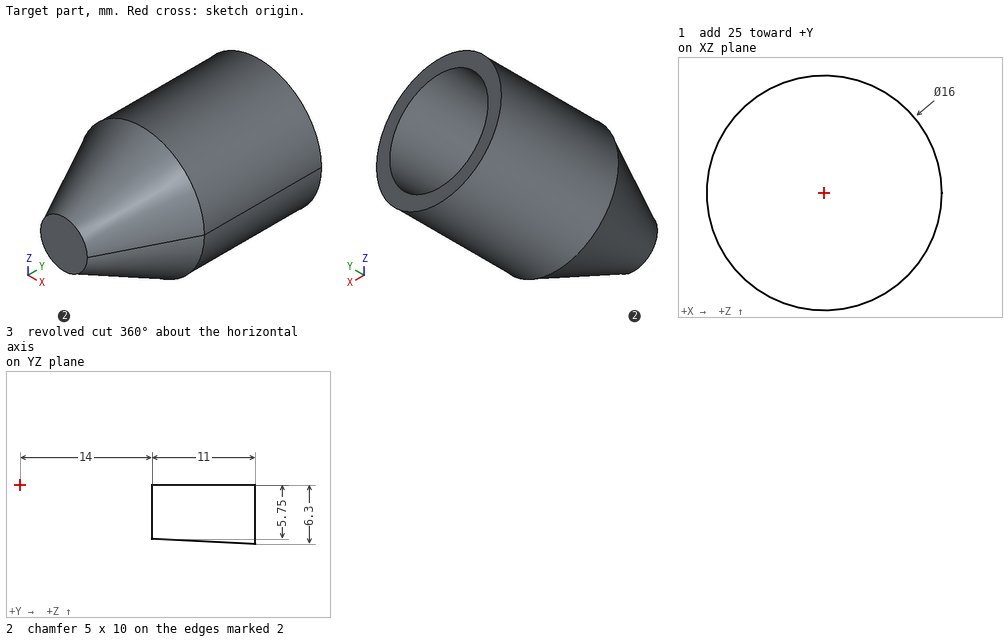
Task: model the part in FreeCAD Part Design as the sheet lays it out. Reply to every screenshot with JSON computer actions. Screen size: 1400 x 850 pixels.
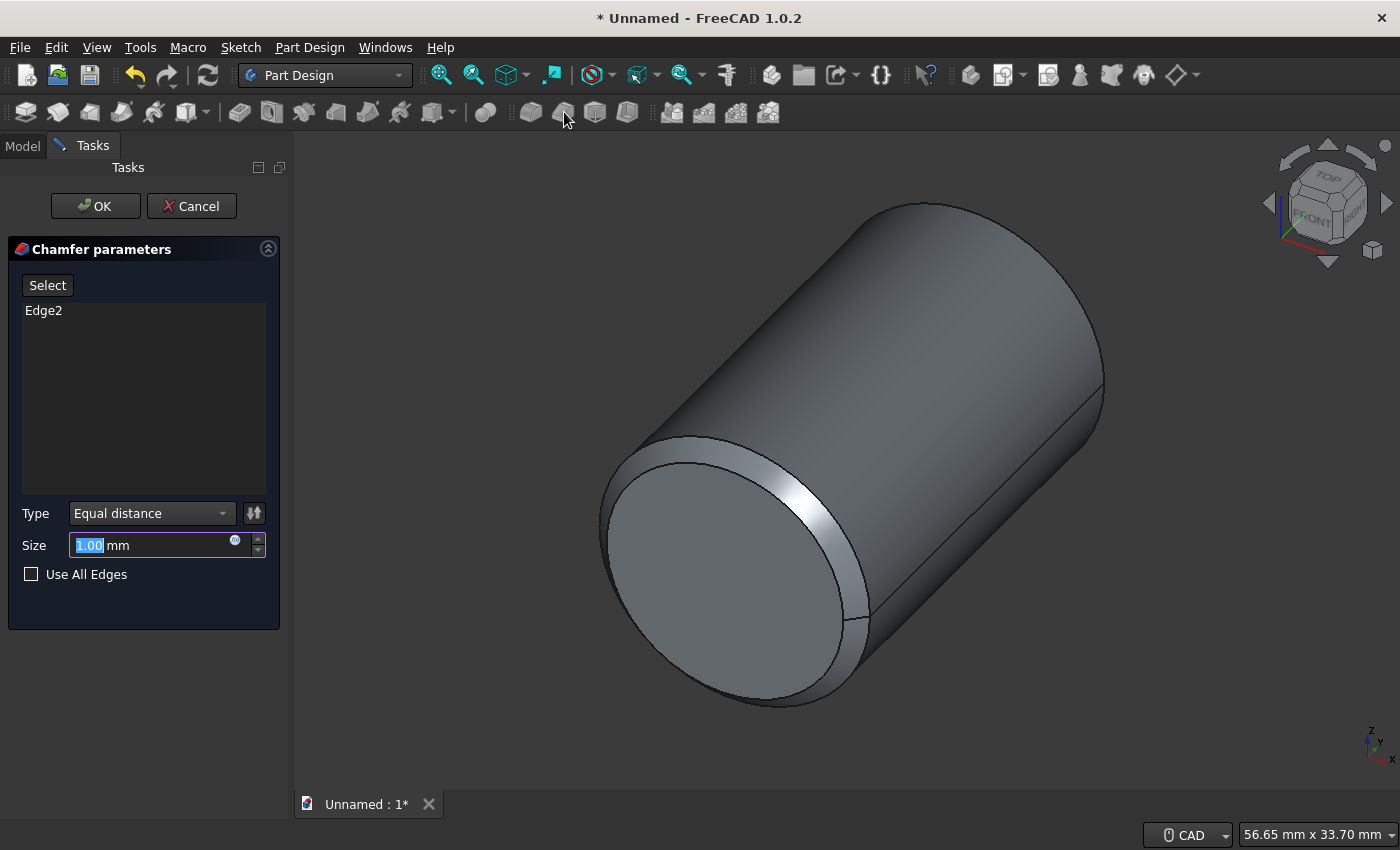
{"action": "type", "text": "5"}
{"action": "key", "text": "Tab"}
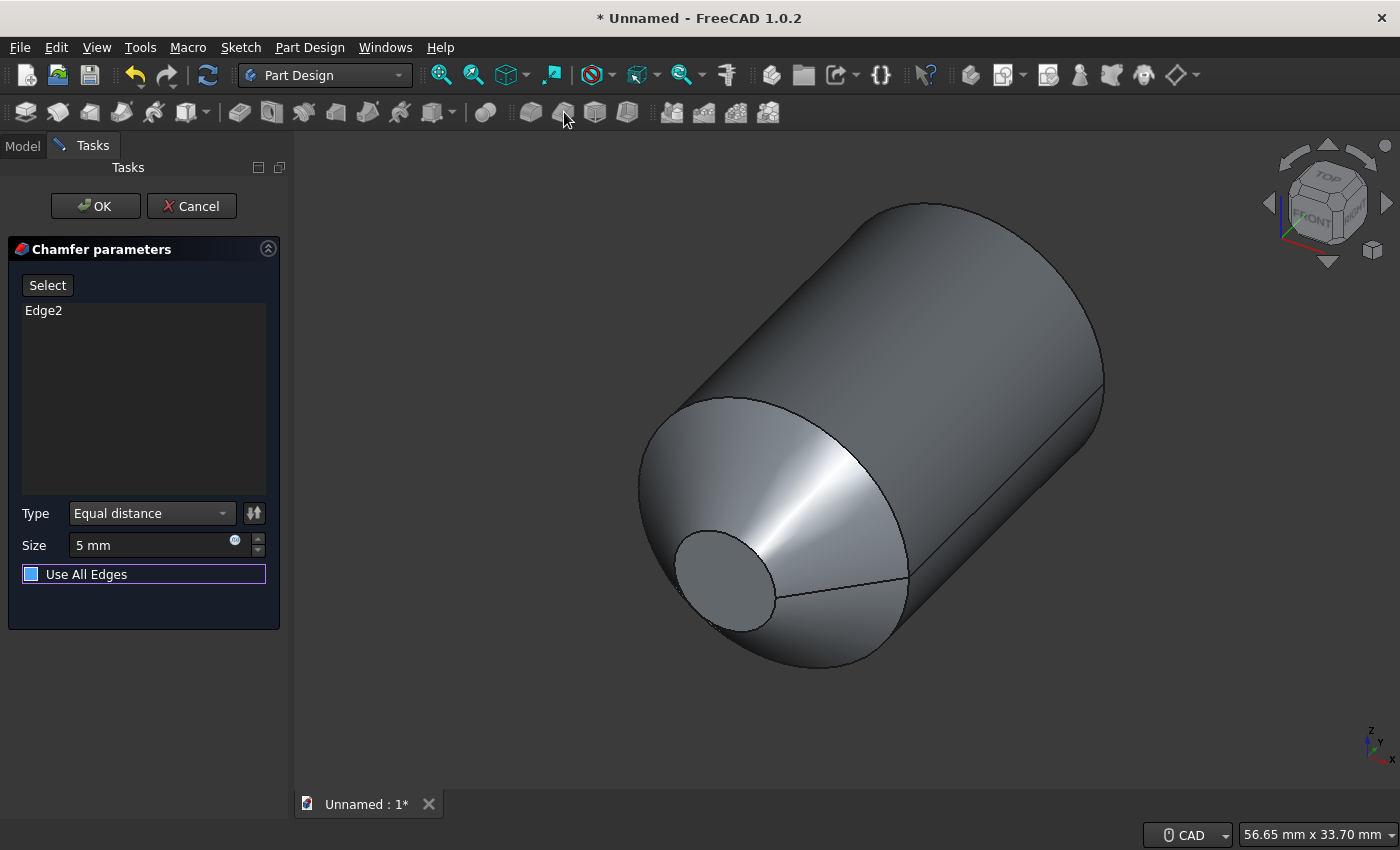
{"action": "left_click", "coordinate": [153, 514]}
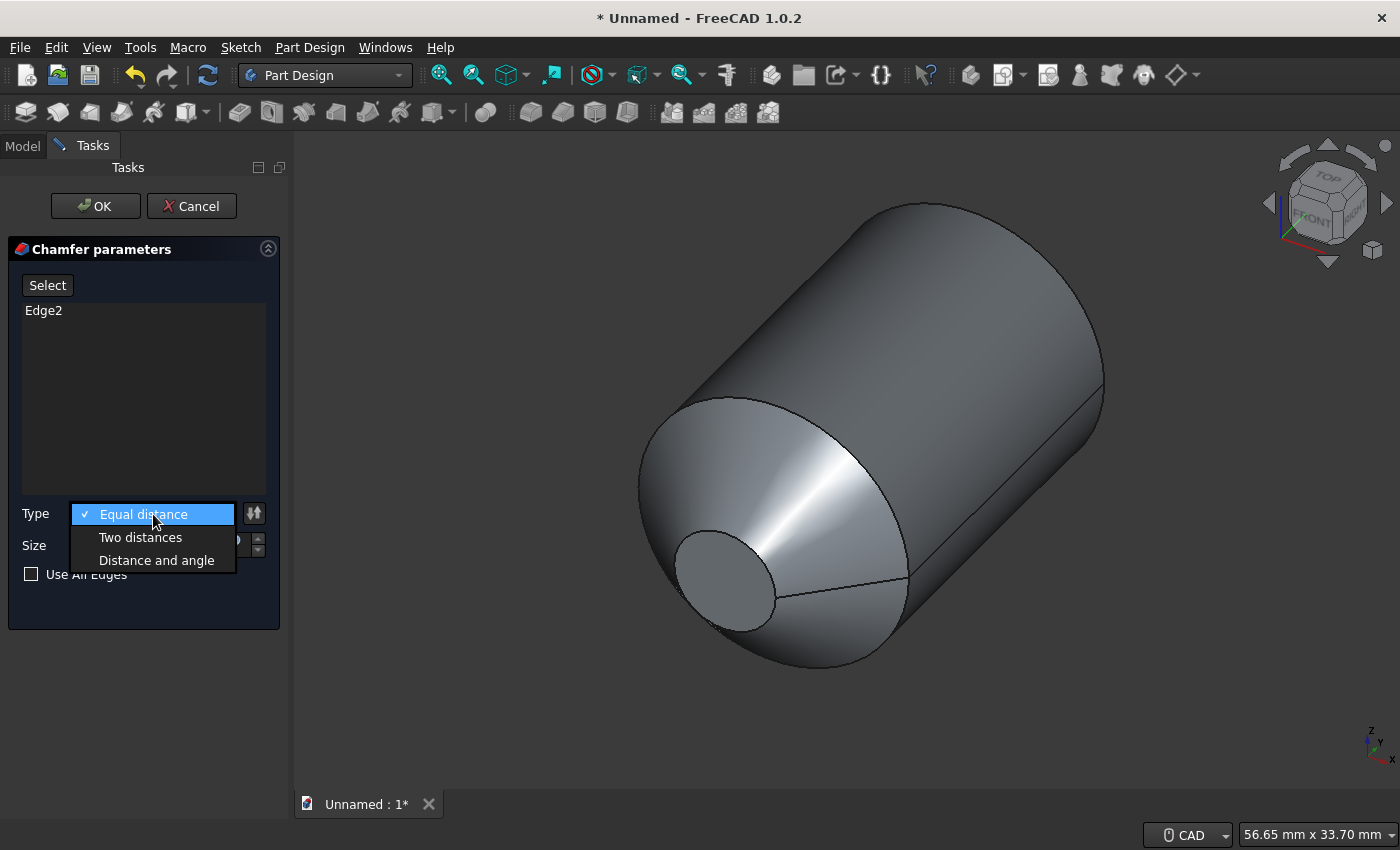
{"action": "left_click", "coordinate": [152, 538]}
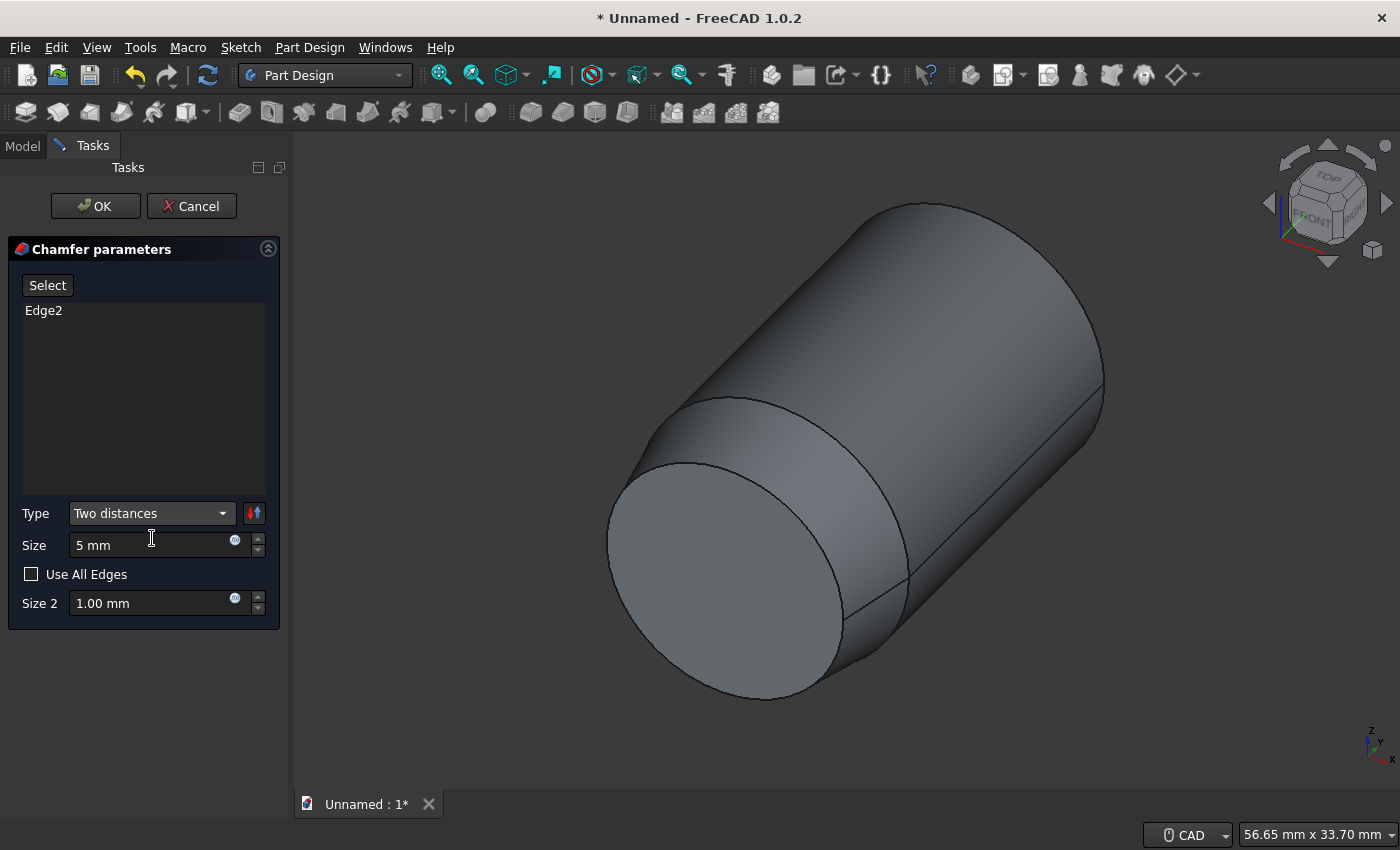
{"action": "triple_click", "coordinate": [160, 603]}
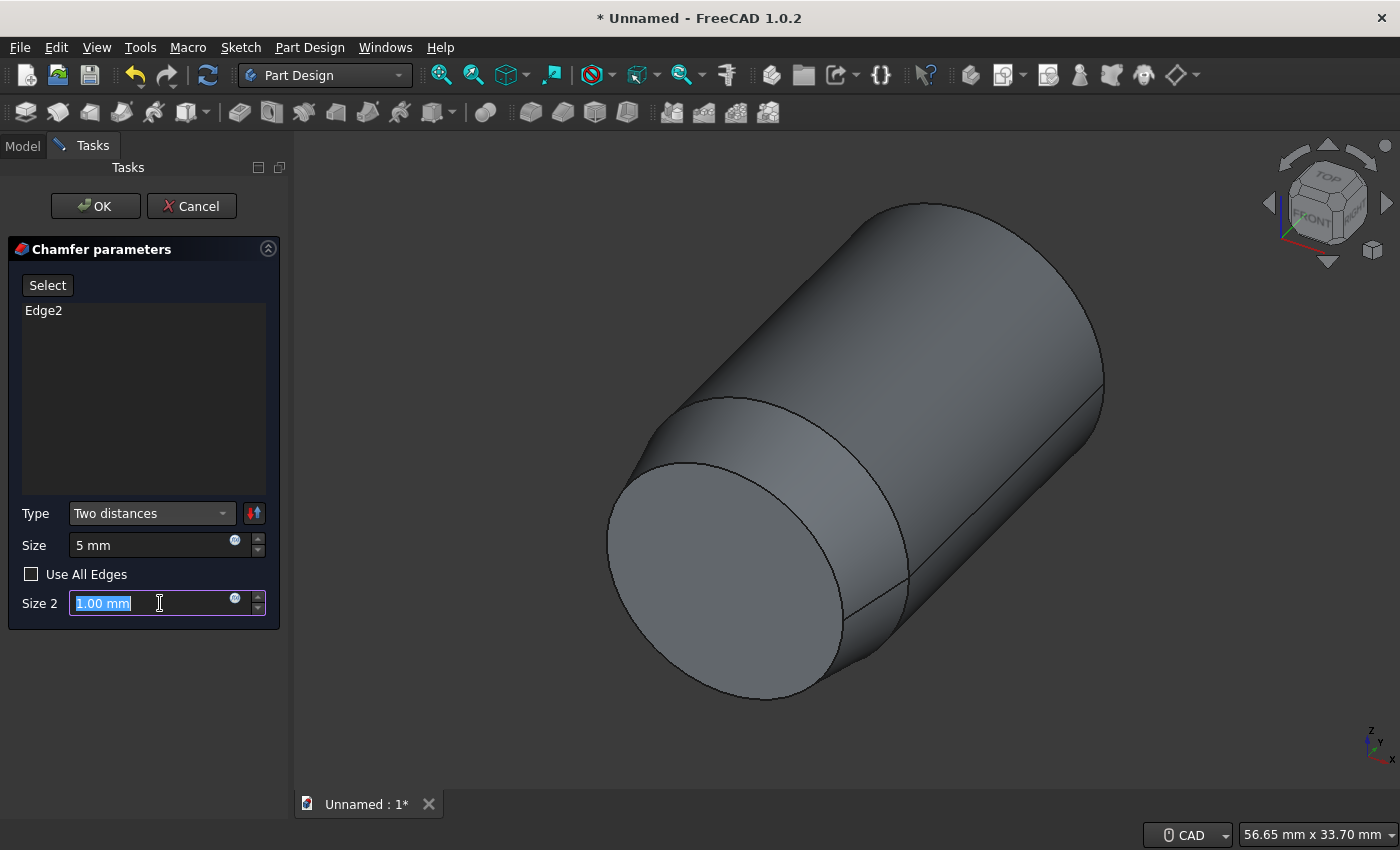
{"action": "type", "text": "10"}
{"action": "key", "text": "Tab"}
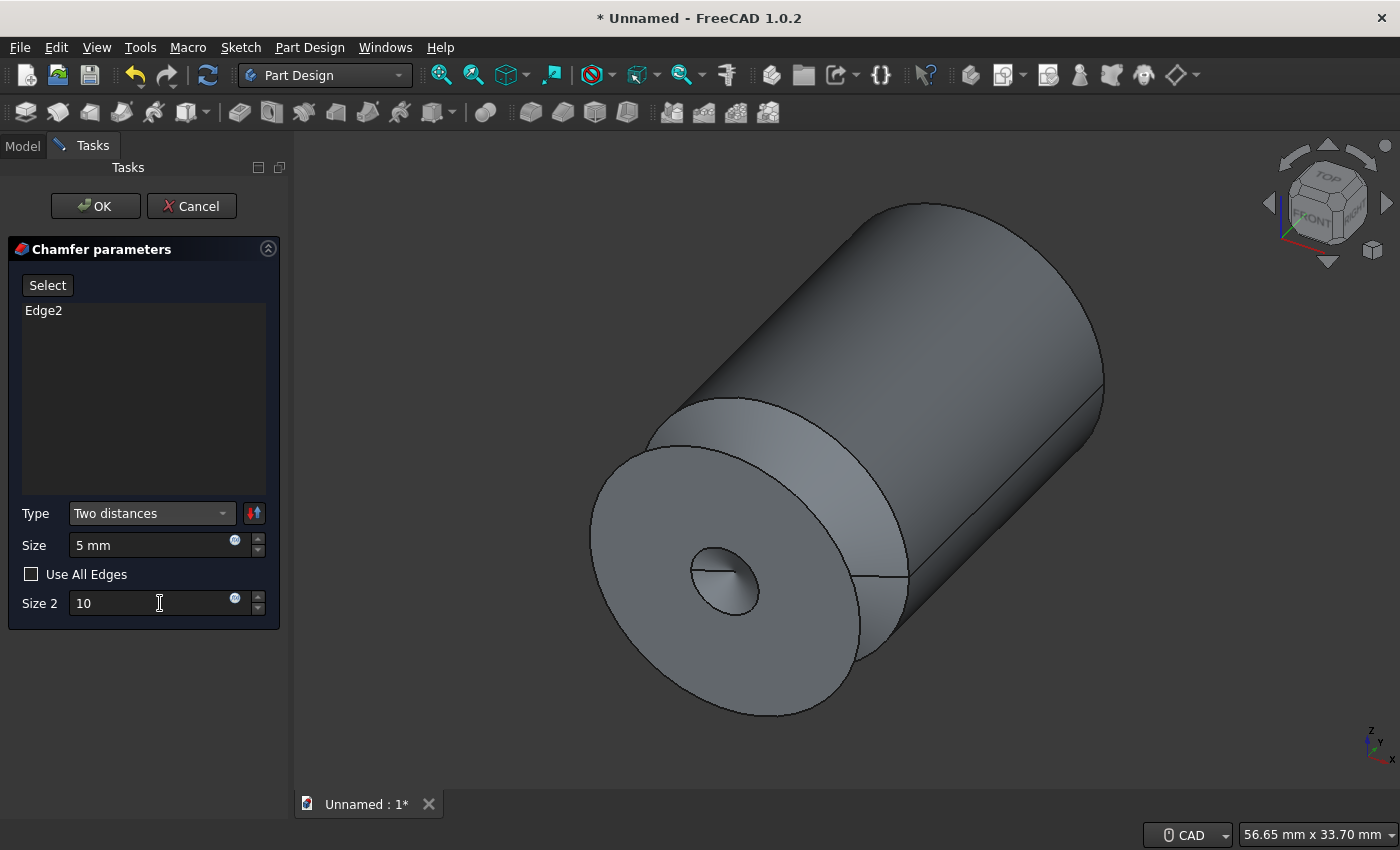
{"action": "left_click", "coordinate": [254, 514]}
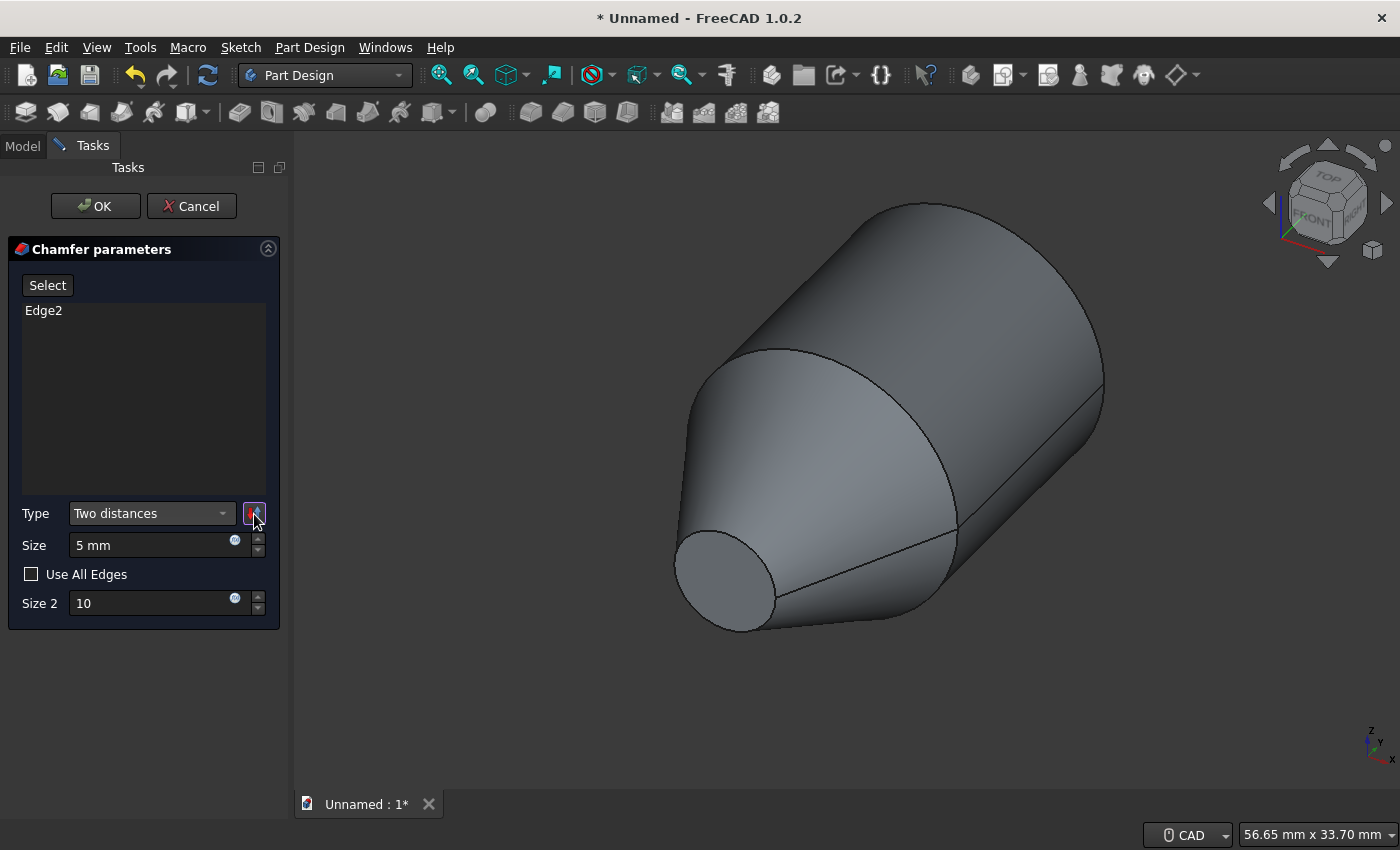
{"action": "left_click", "coordinate": [96, 206]}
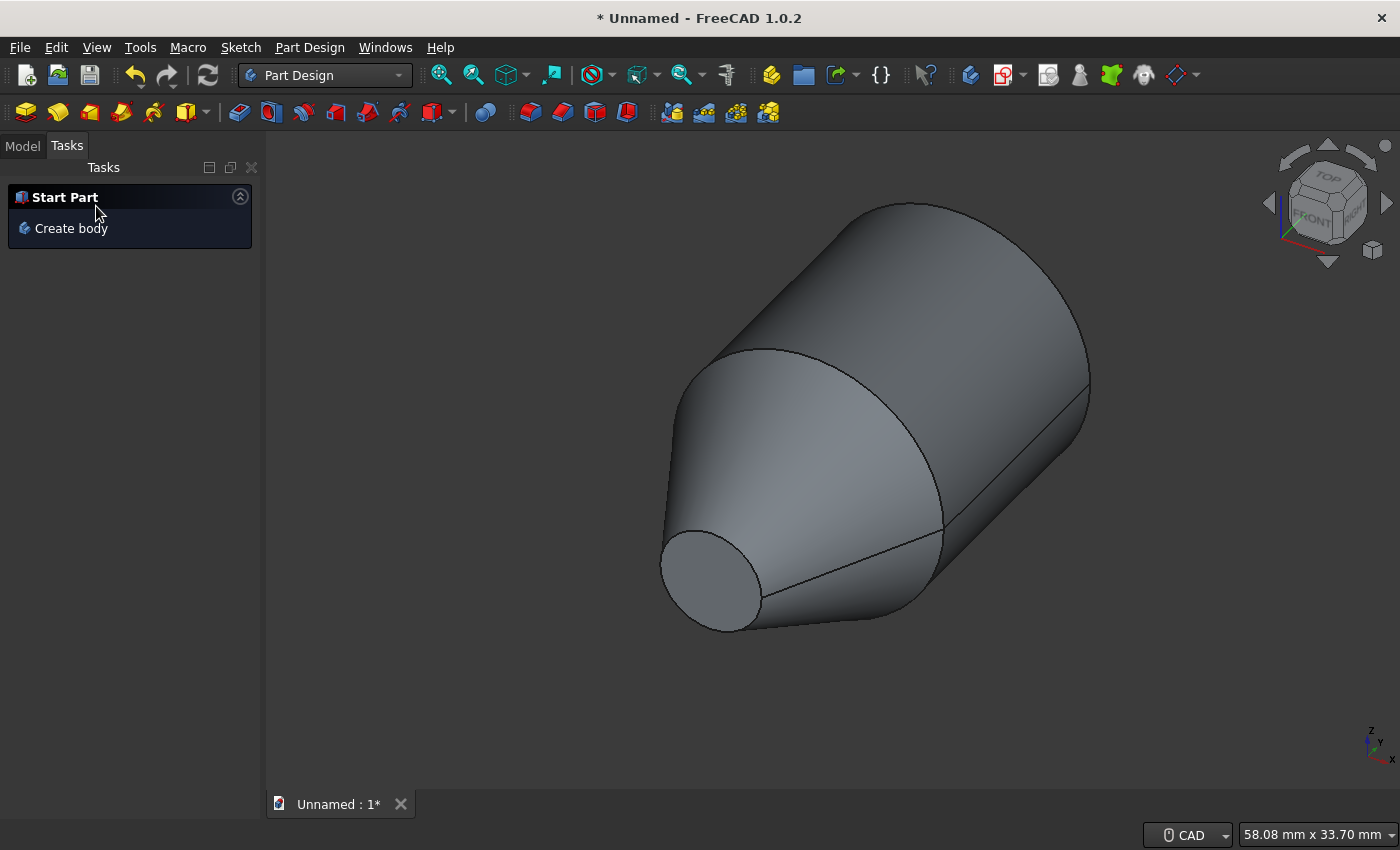
{"action": "left_click", "coordinate": [1004, 76]}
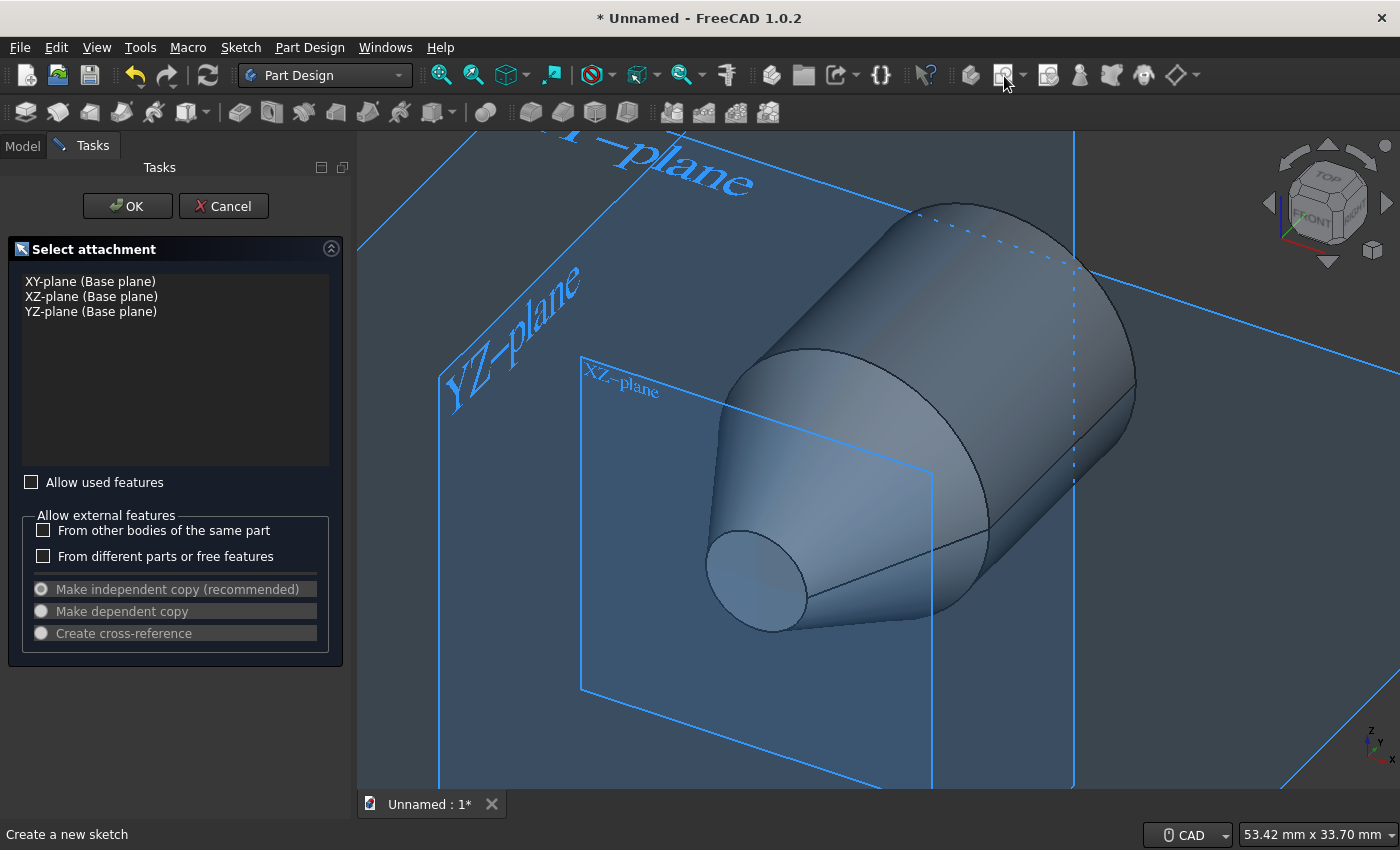
{"action": "left_click", "coordinate": [82, 312]}